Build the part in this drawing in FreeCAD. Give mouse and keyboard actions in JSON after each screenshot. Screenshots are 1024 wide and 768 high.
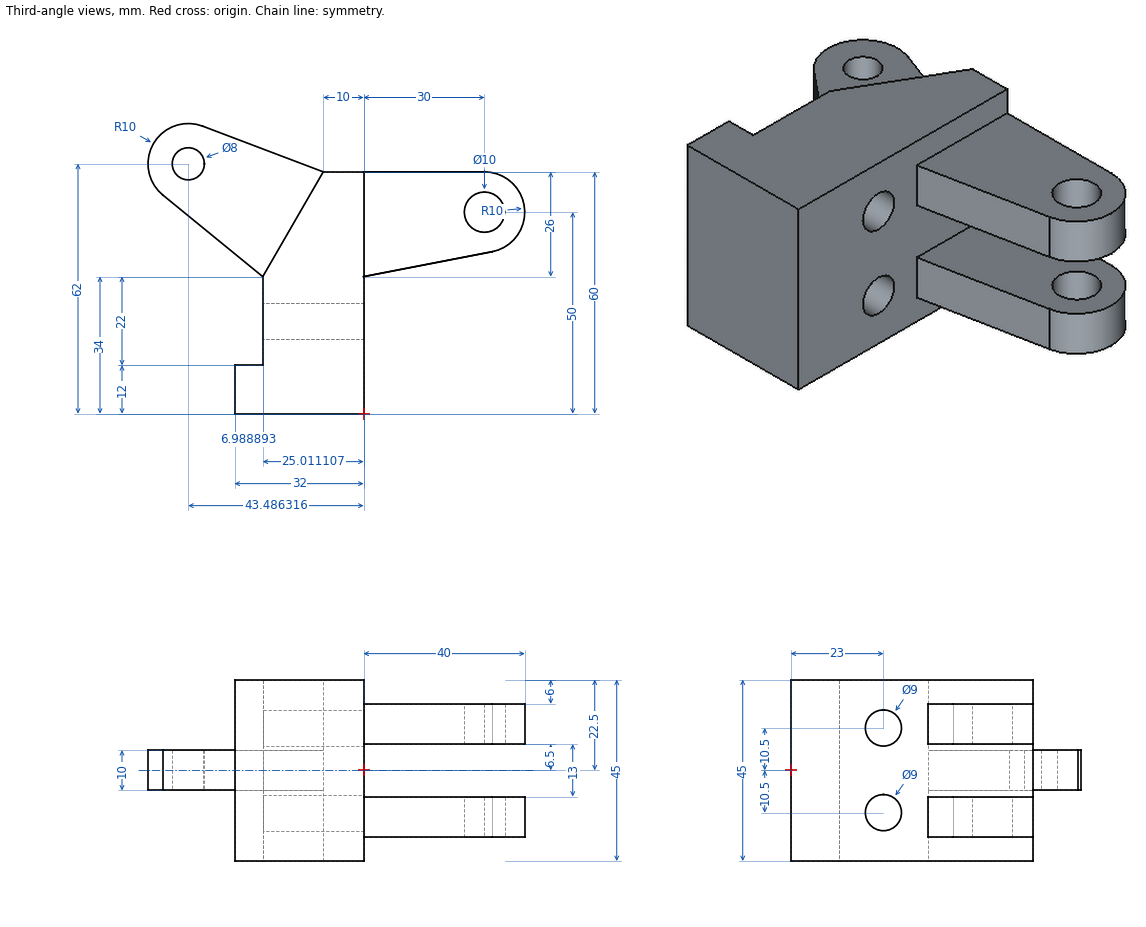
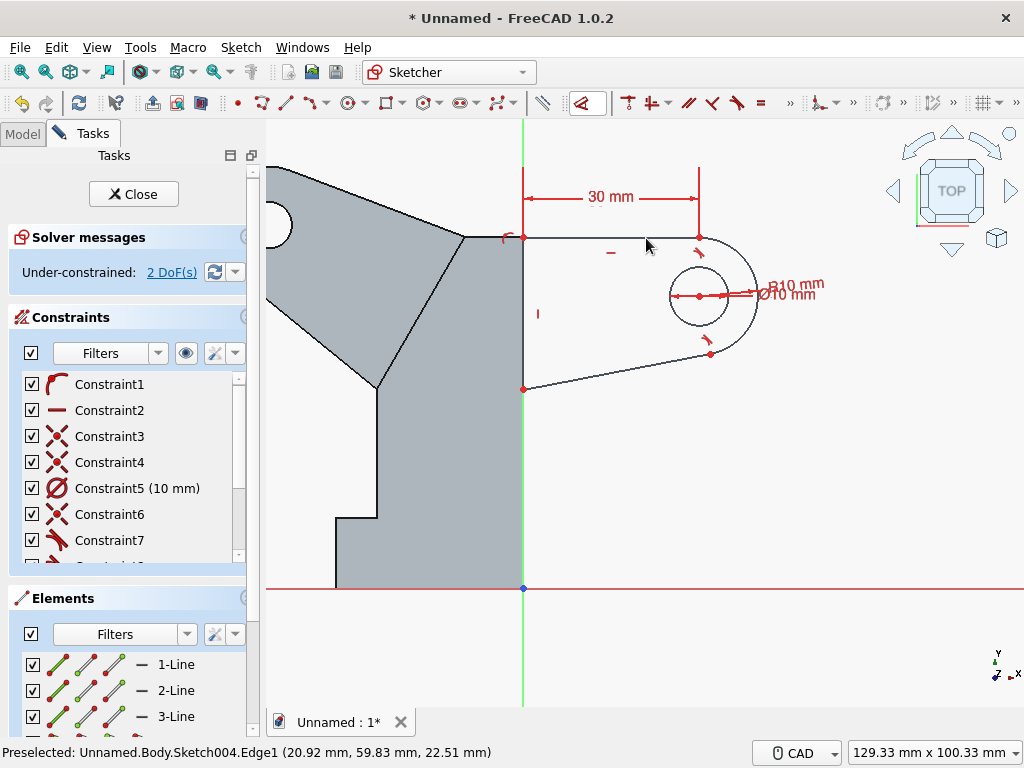
{"action": "left_click", "coordinate": [523, 283]}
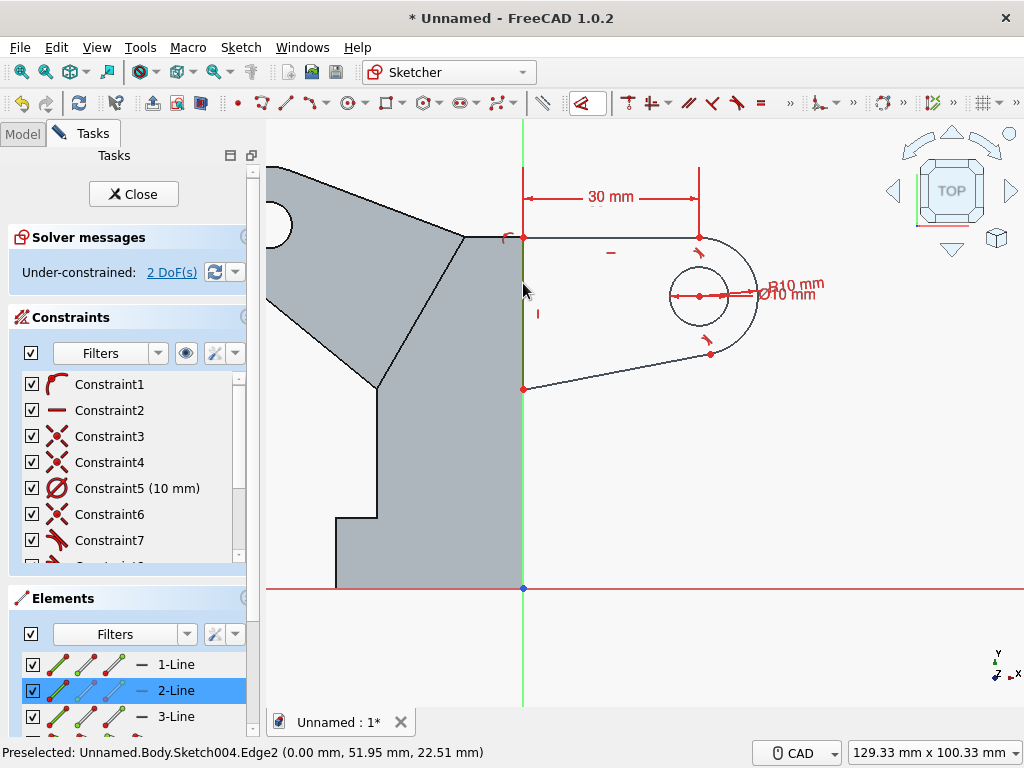
{"action": "key", "text": "i"}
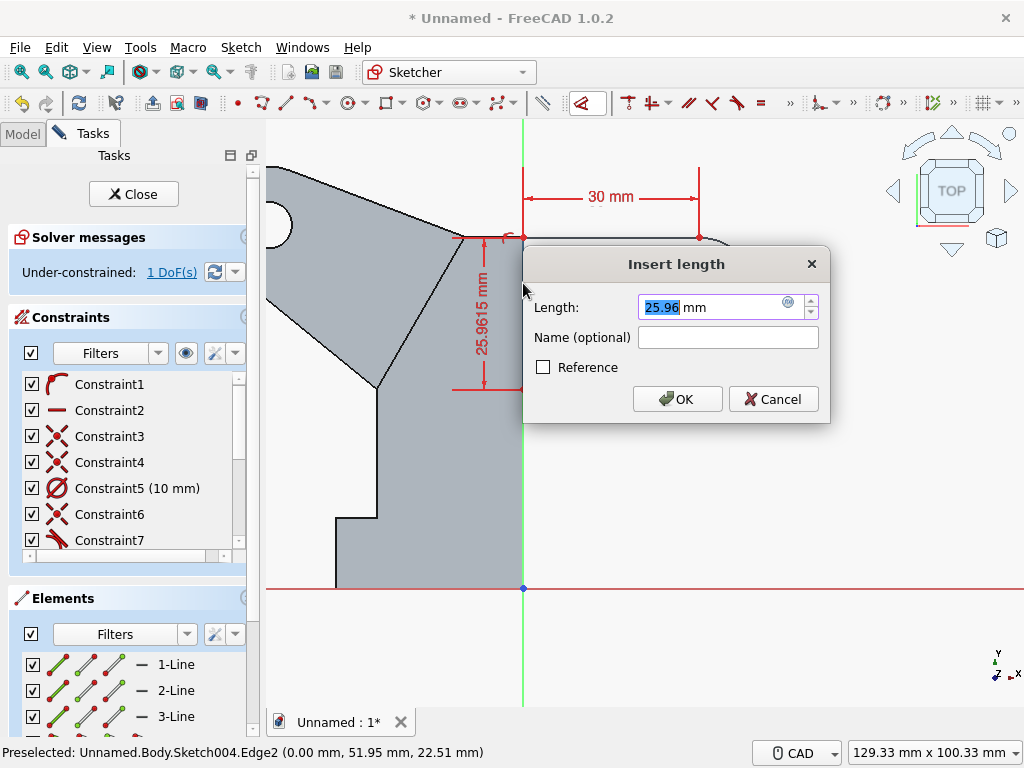
{"action": "type", "text": "26"}
{"action": "key", "text": "Return"}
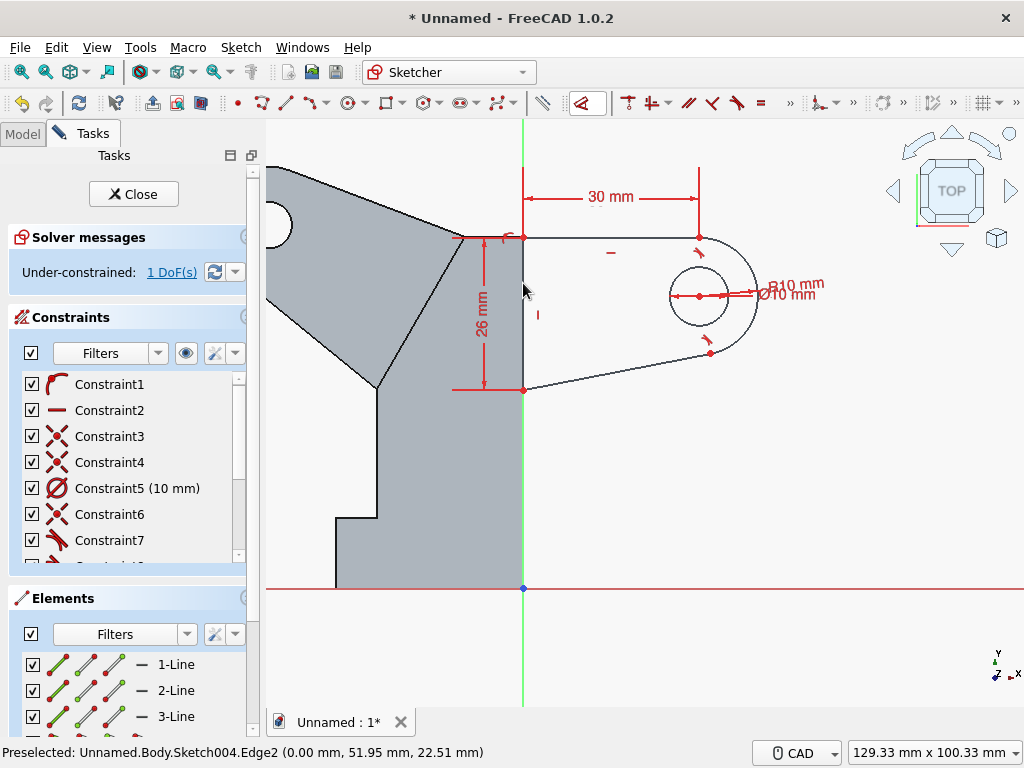
{"action": "left_click", "coordinate": [699, 296]}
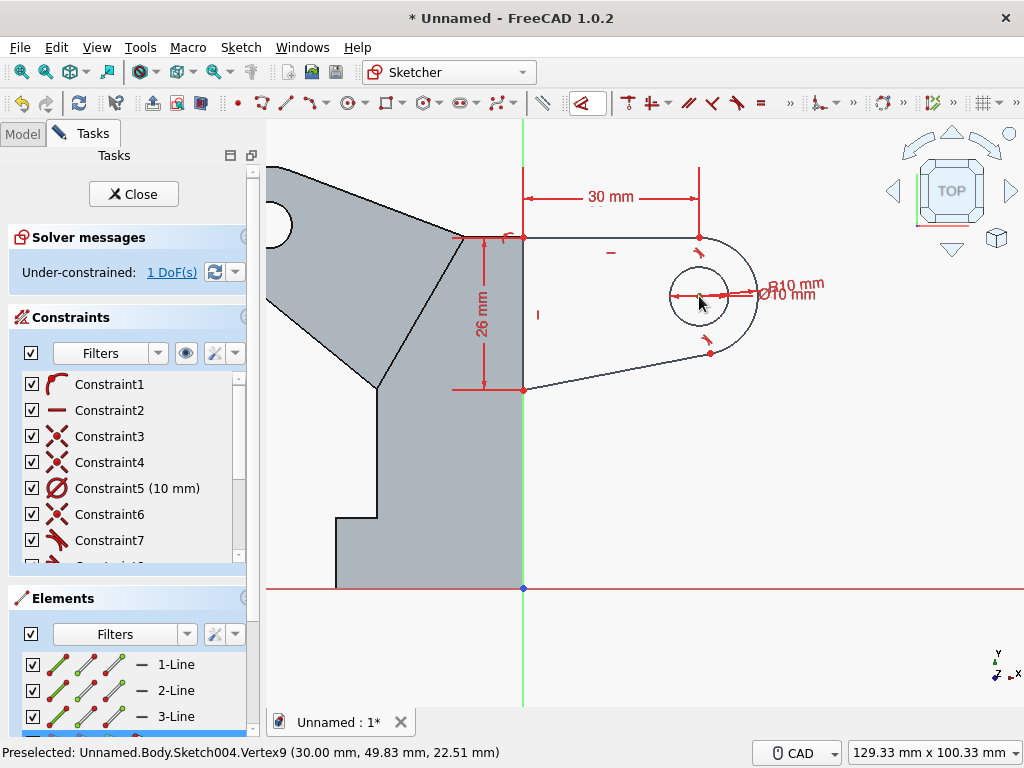
{"action": "key", "text": "i"}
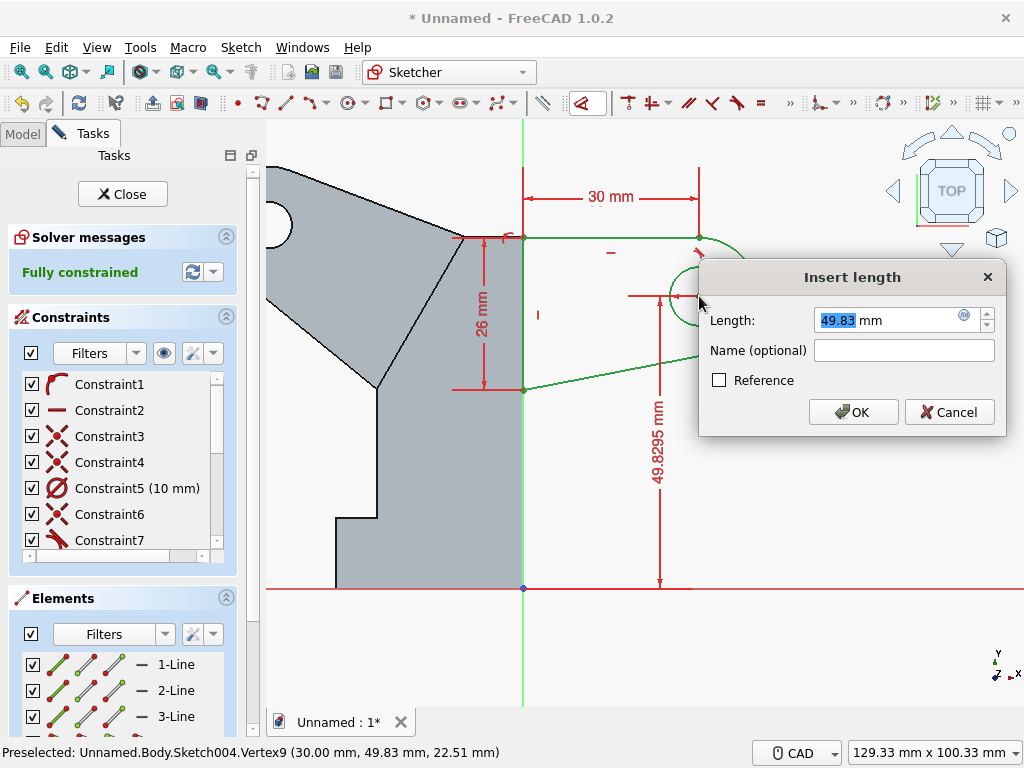
{"action": "type", "text": "50"}
{"action": "key", "text": "Return"}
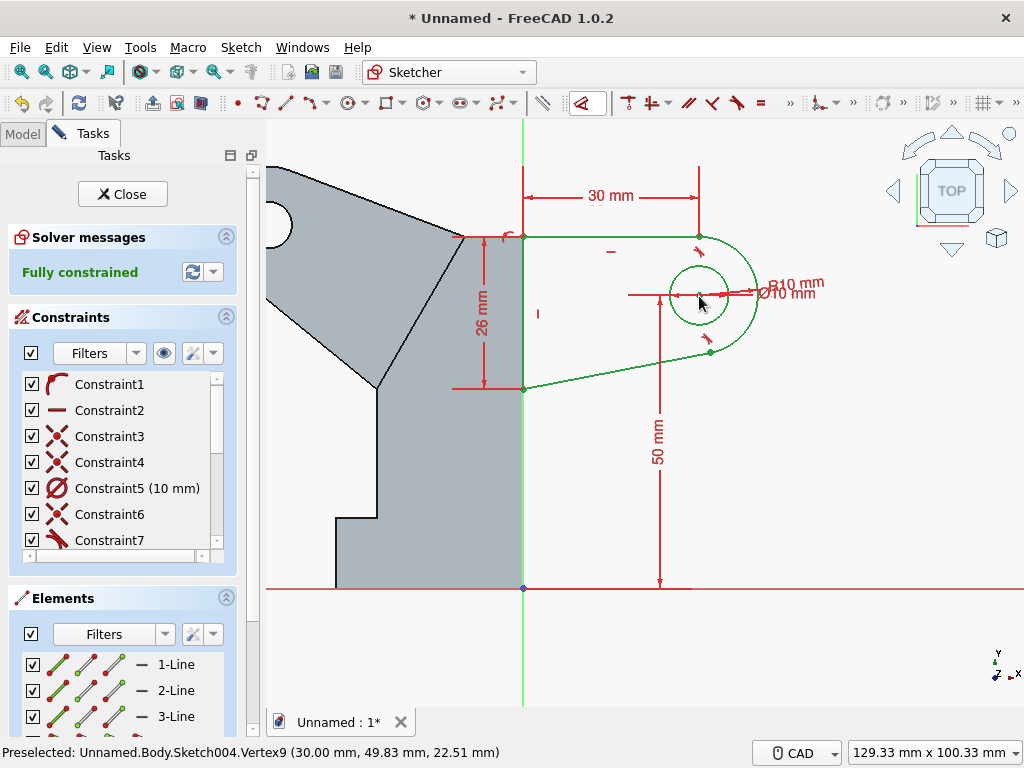
{"action": "left_click", "coordinate": [123, 194]}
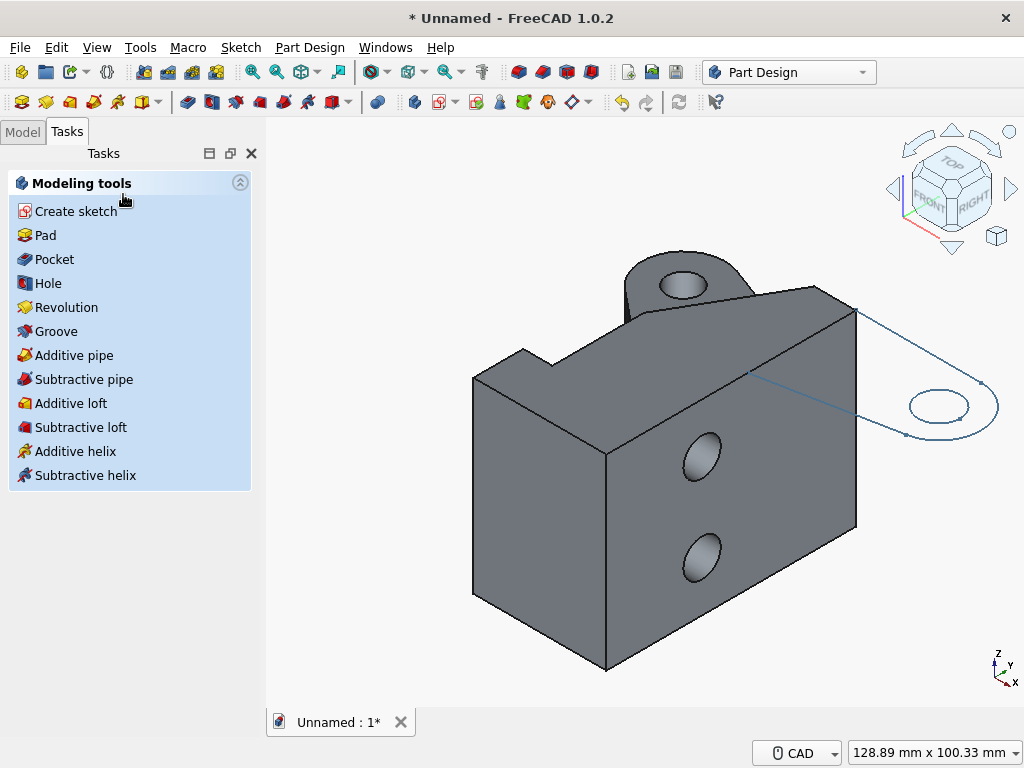
{"action": "left_click", "coordinate": [22, 102]}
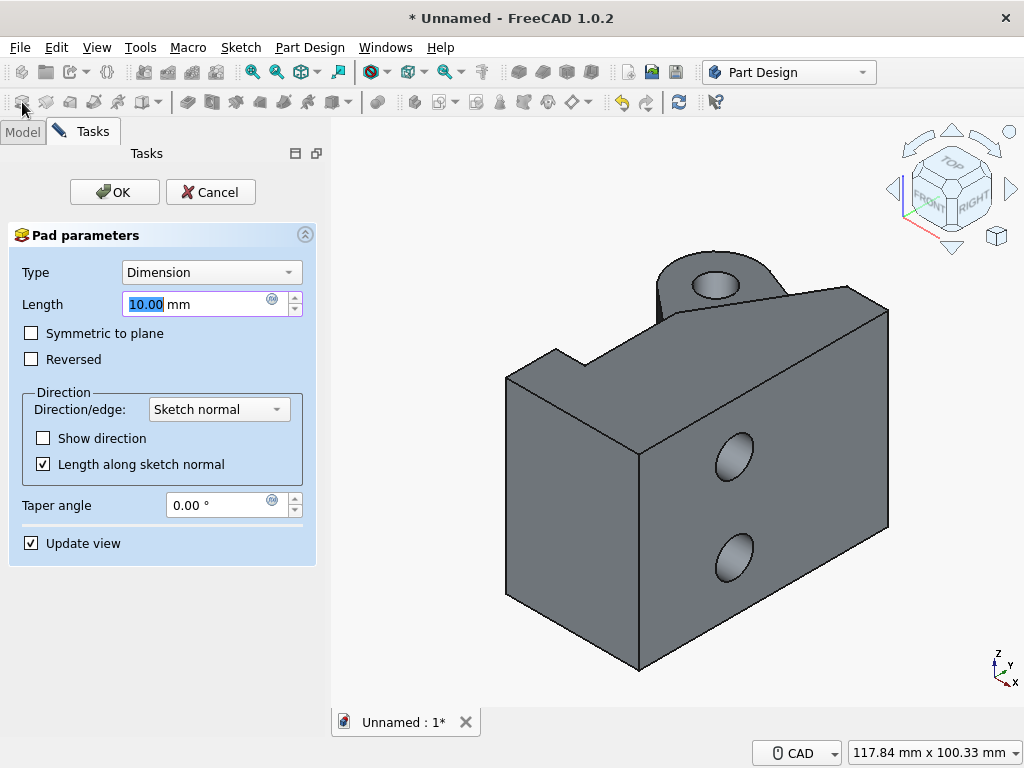
{"action": "type", "text": "45"}
{"action": "key", "text": "Tab"}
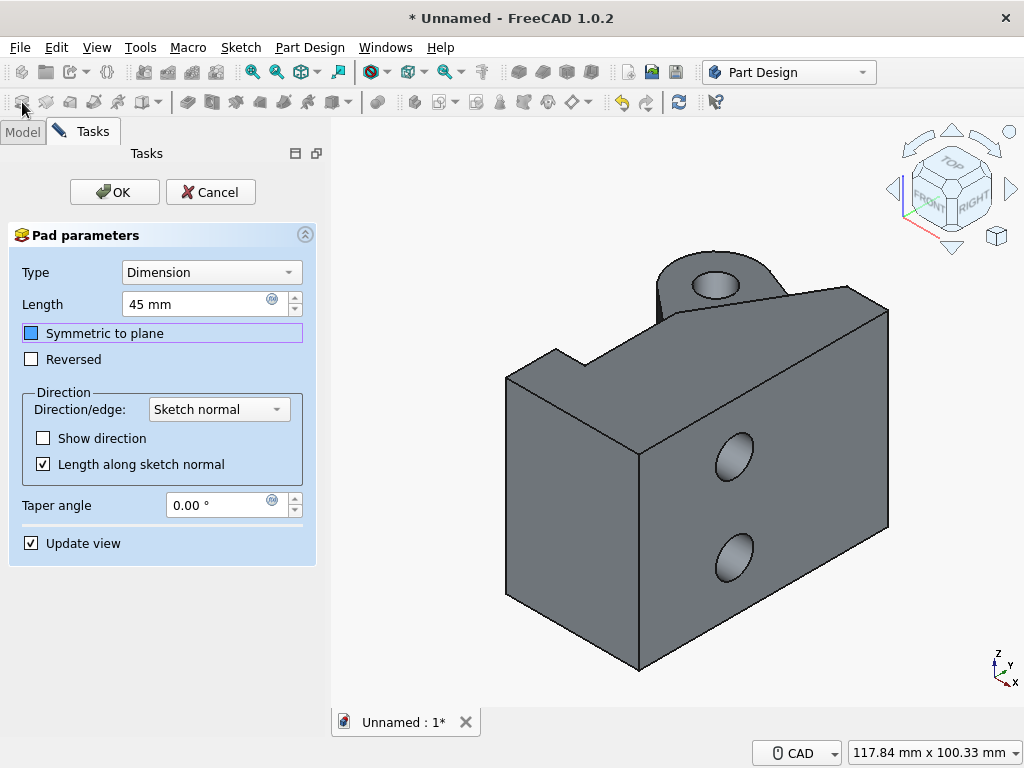
{"action": "left_click", "coordinate": [30, 359]}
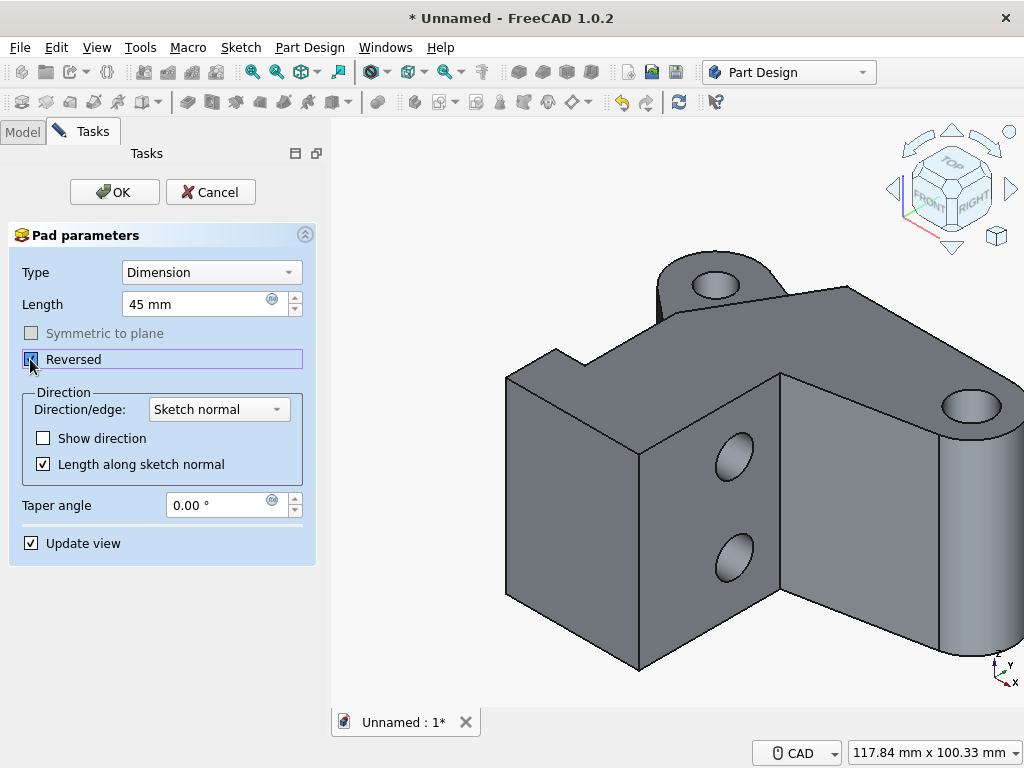
{"action": "left_click", "coordinate": [115, 192]}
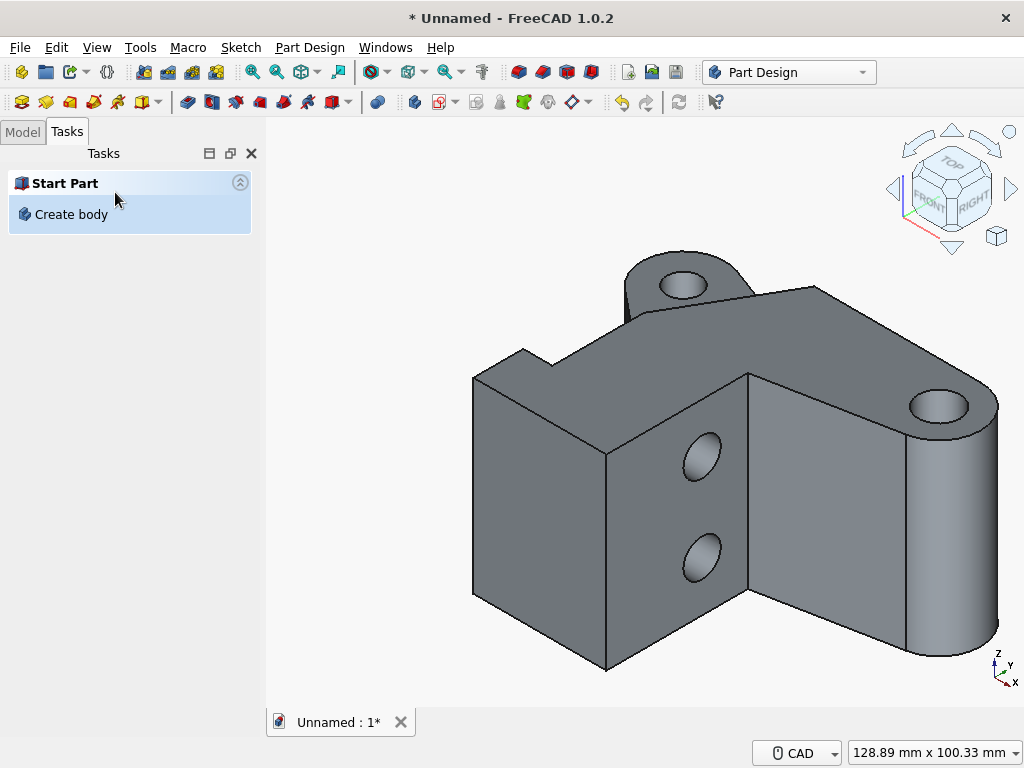
{"action": "left_click", "coordinate": [254, 72]}